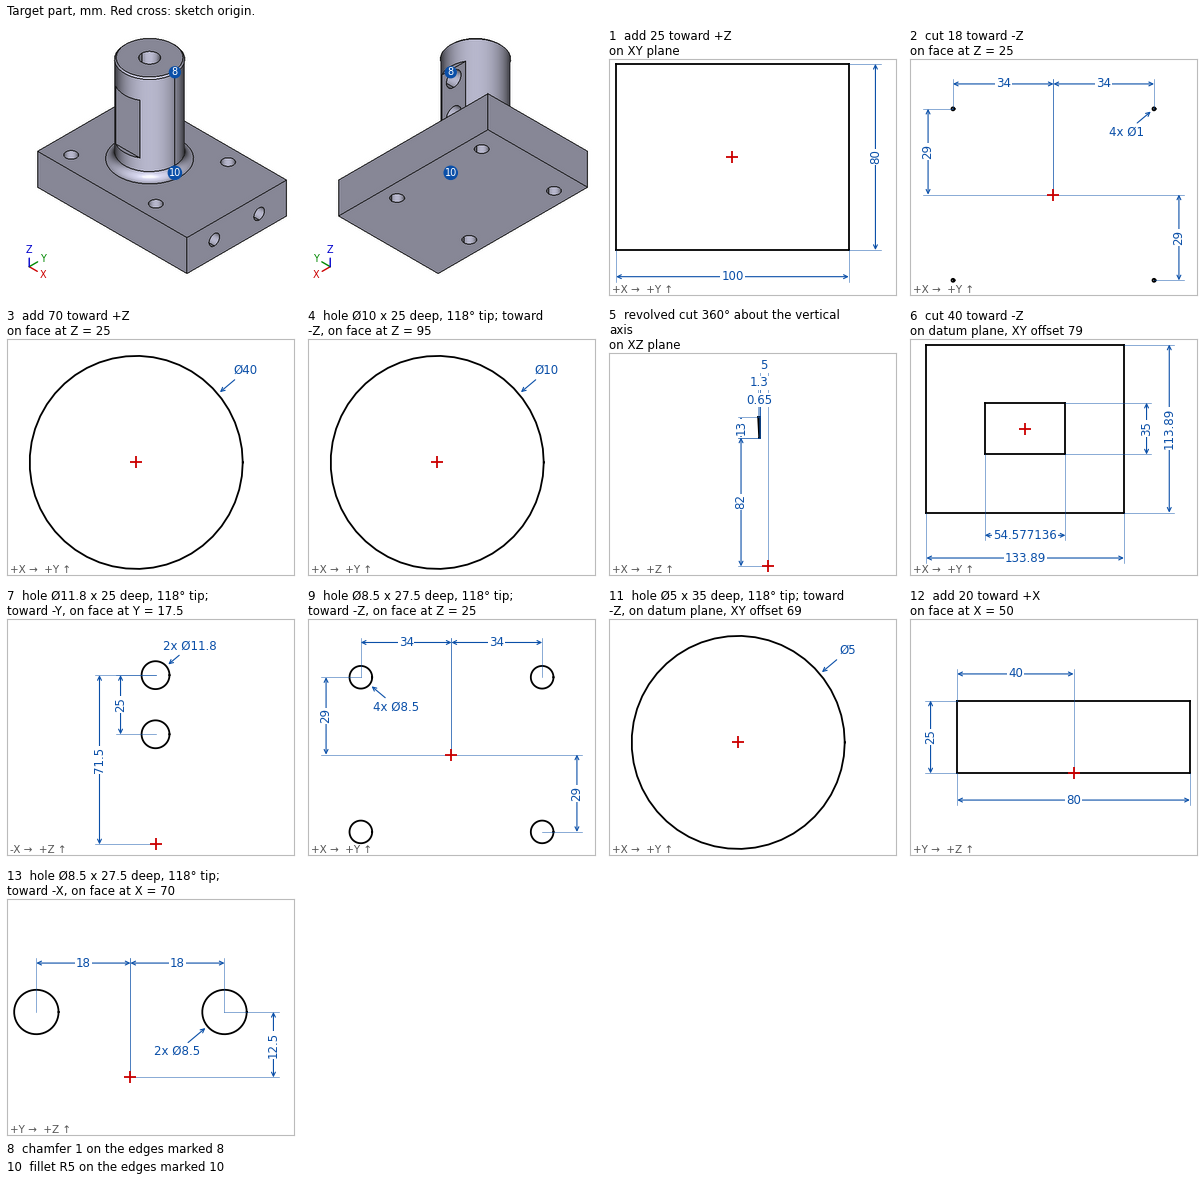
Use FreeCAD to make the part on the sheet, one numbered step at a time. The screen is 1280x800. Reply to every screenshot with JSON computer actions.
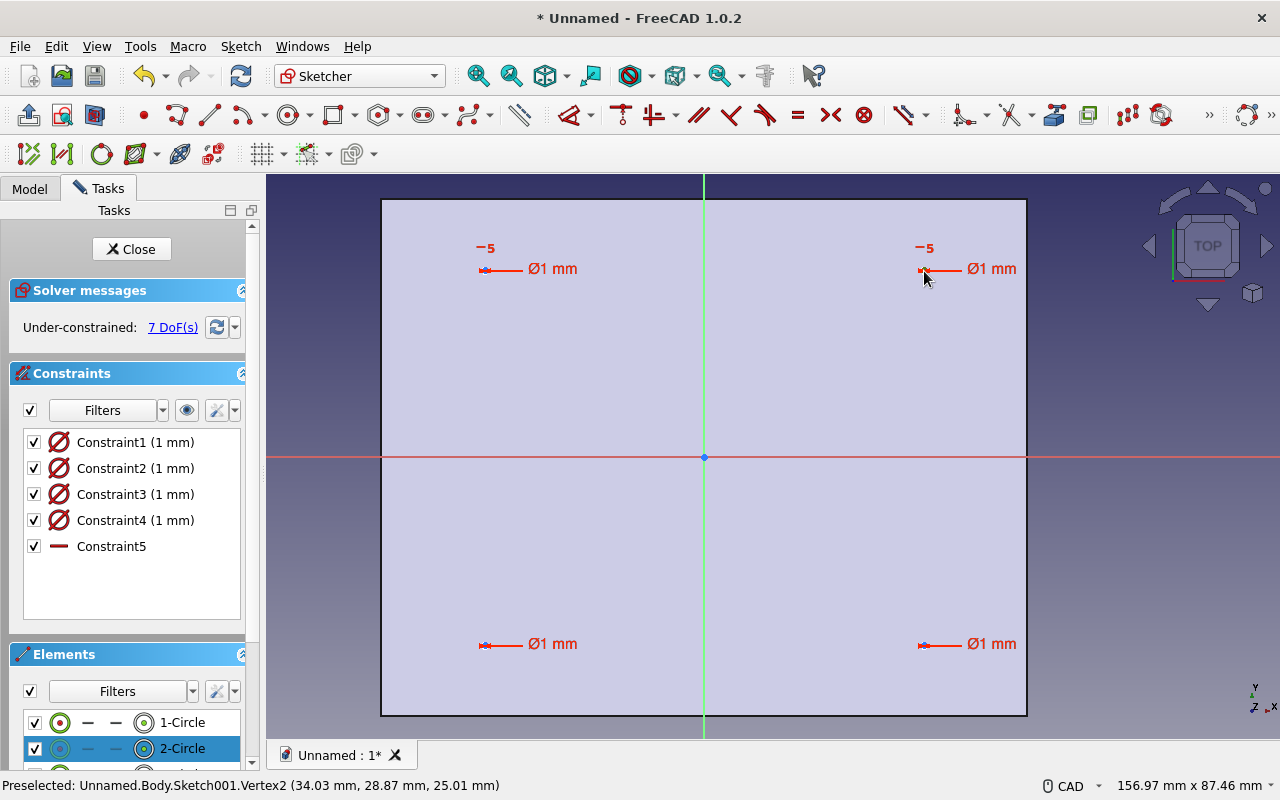
{"action": "left_click", "coordinate": [924, 646]}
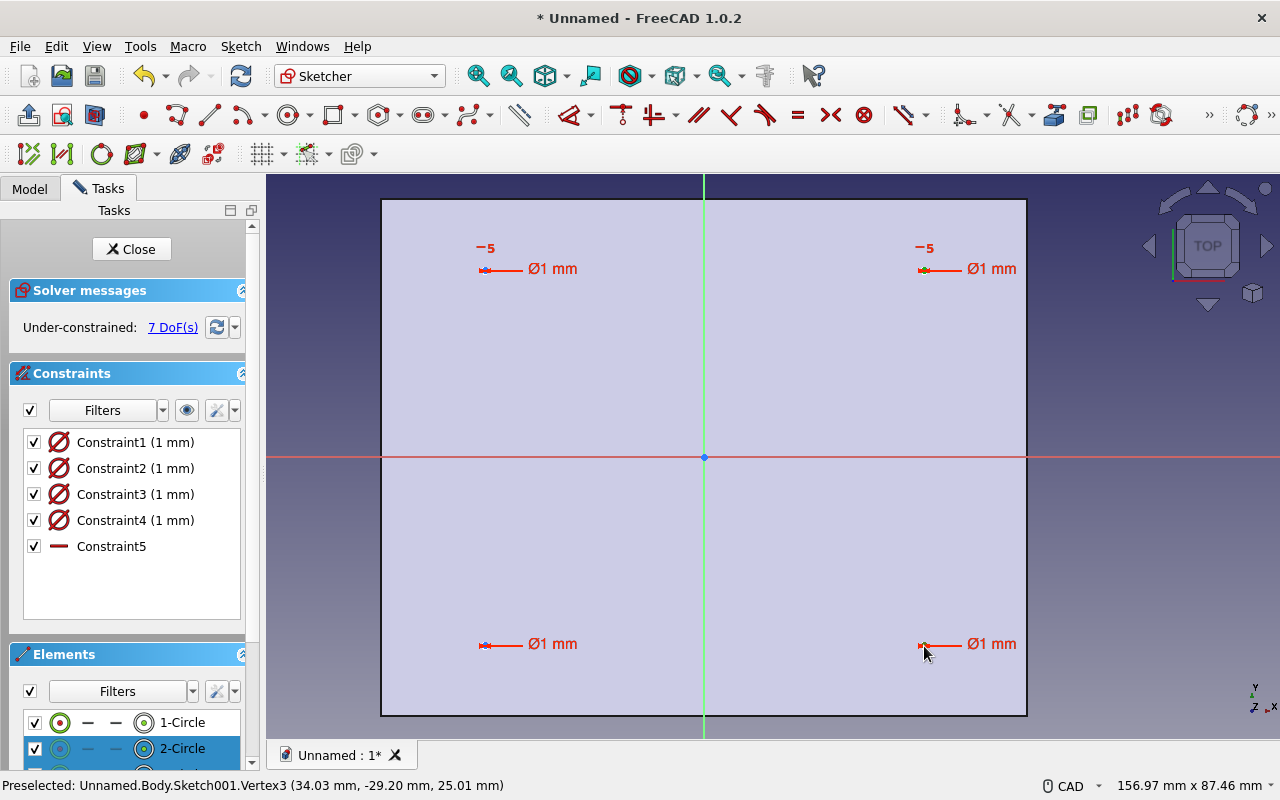
{"action": "key", "text": "v"}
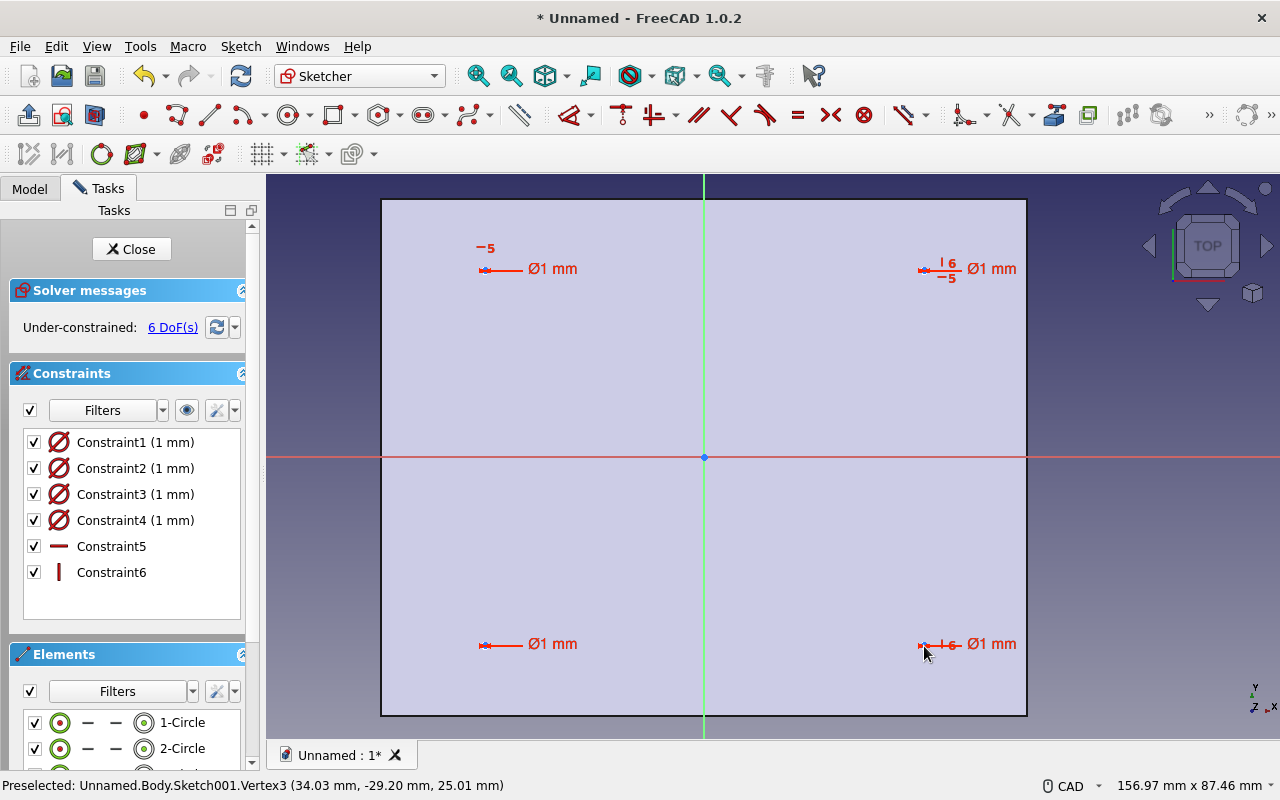
{"action": "left_click", "coordinate": [485, 271]}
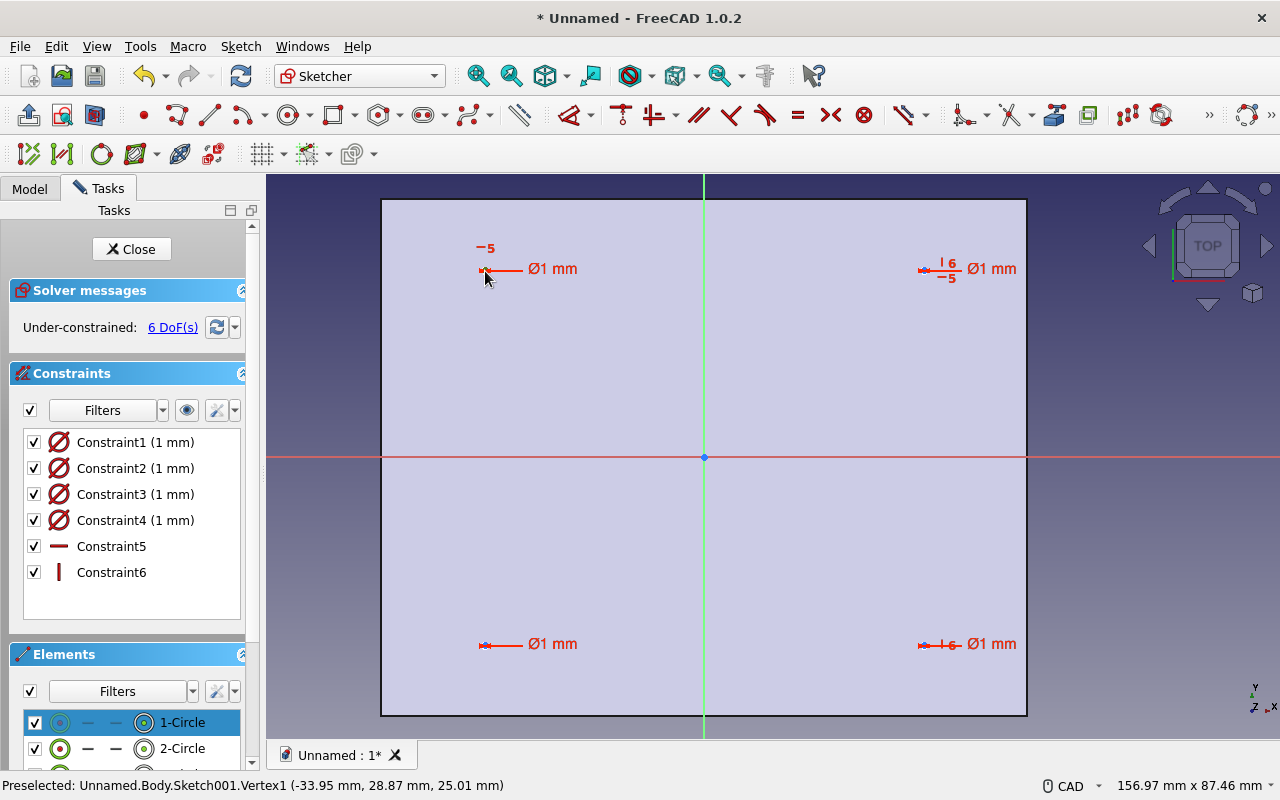
{"action": "left_click", "coordinate": [485, 646]}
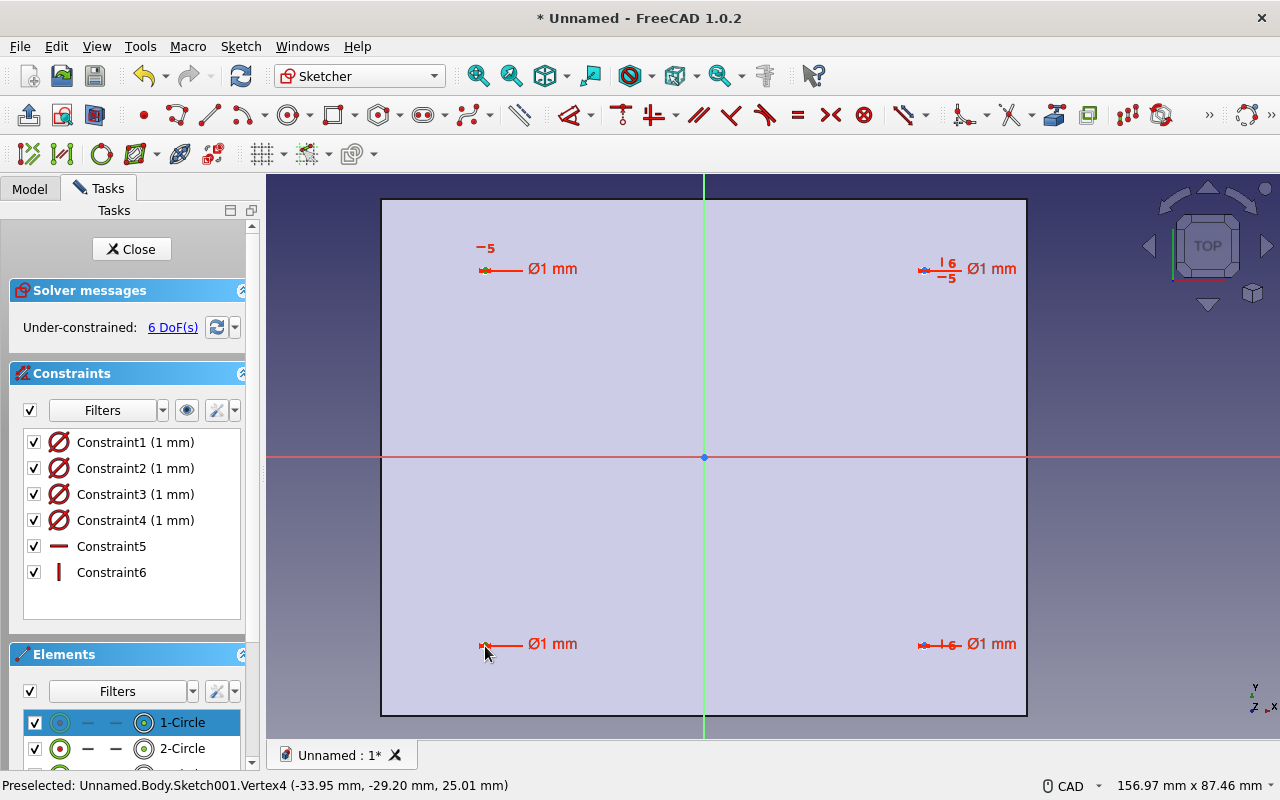
{"action": "key", "text": "v"}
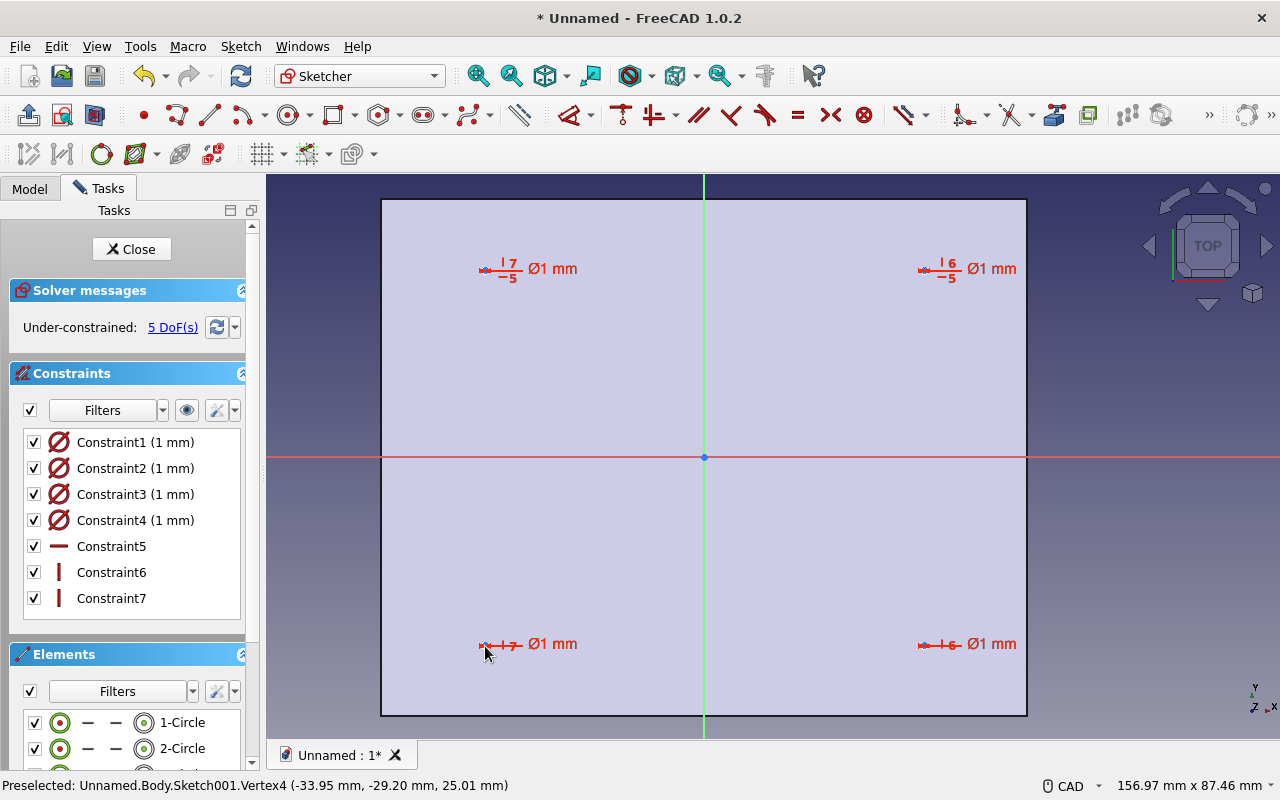
{"action": "left_click", "coordinate": [924, 646]}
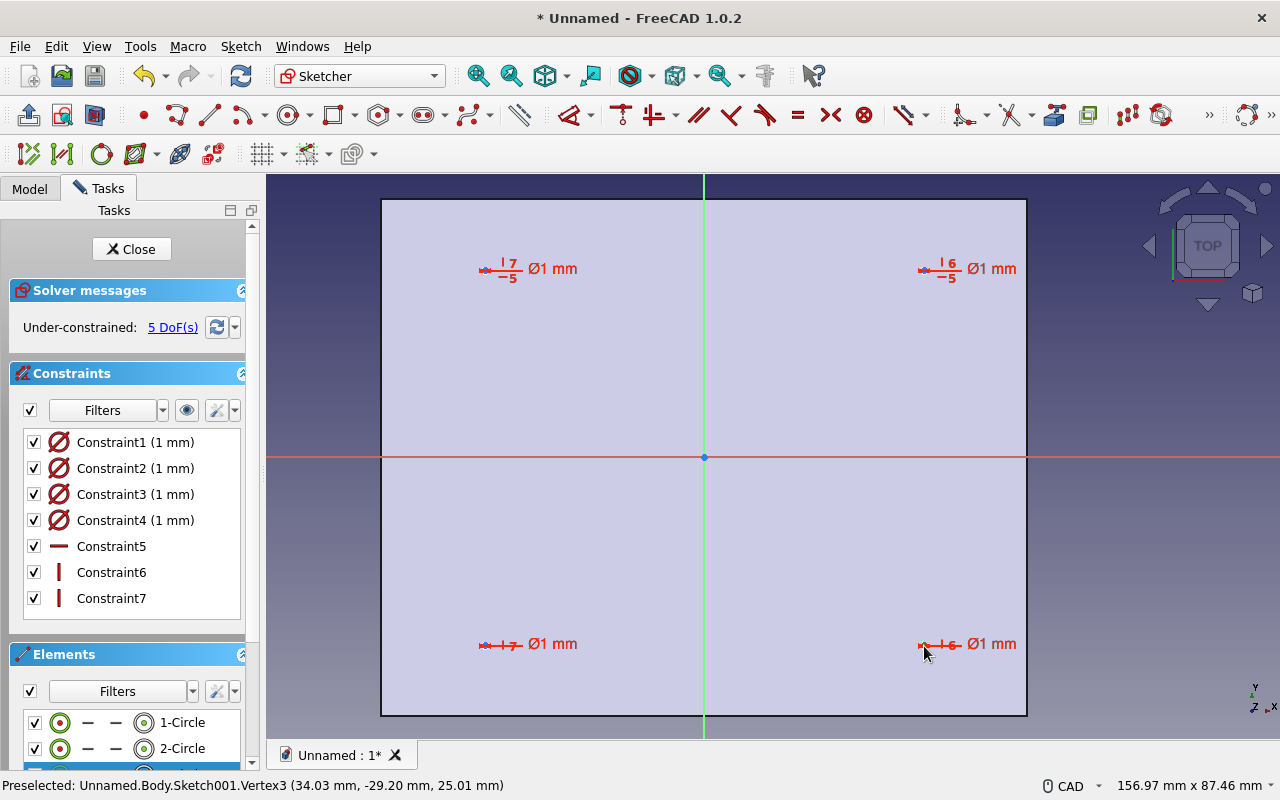
{"action": "left_click", "coordinate": [485, 646]}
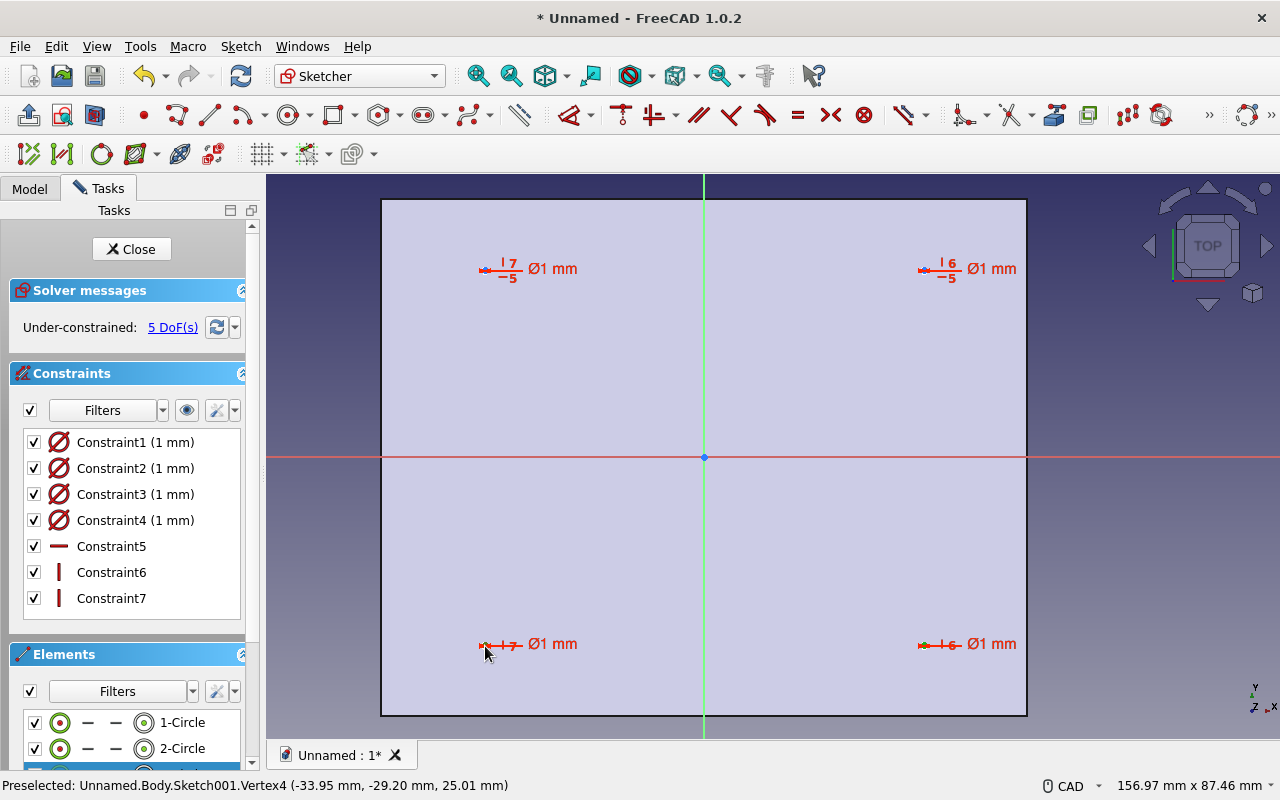
{"action": "key", "text": "h"}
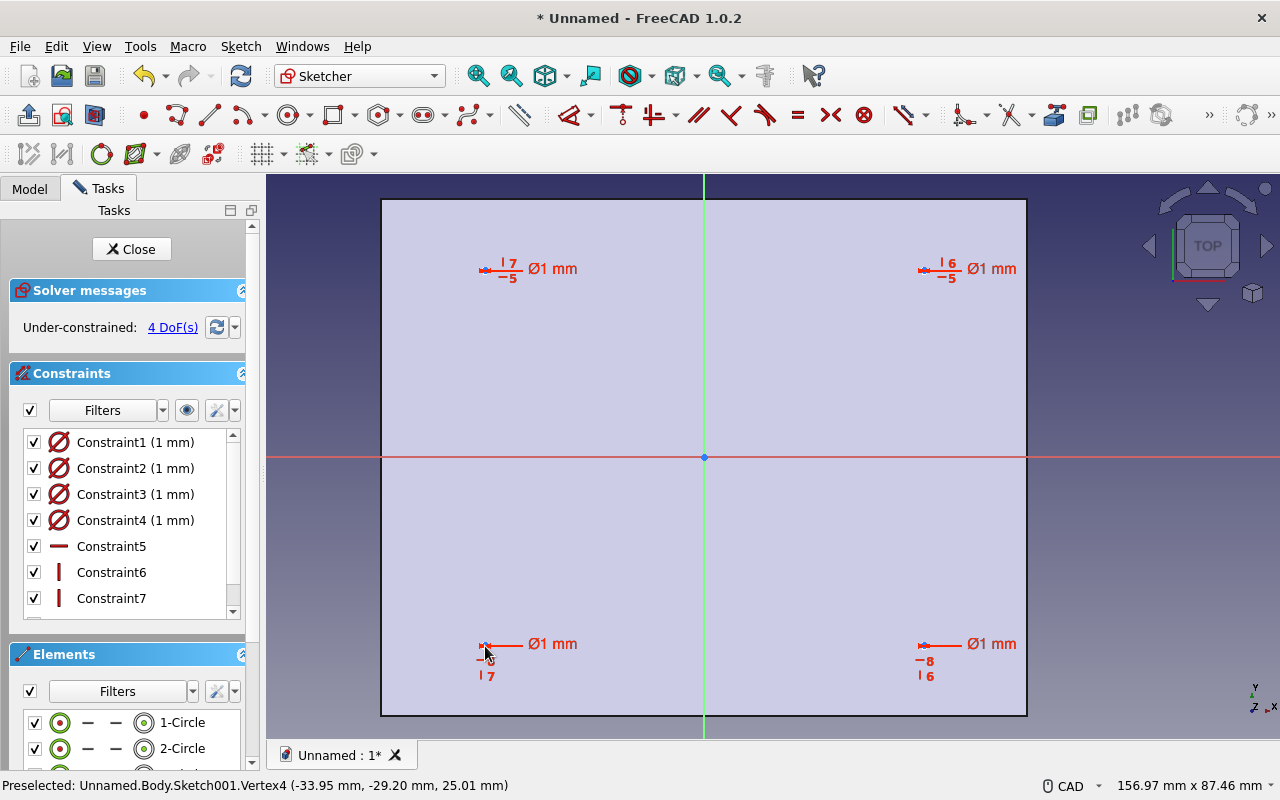
{"action": "left_click", "coordinate": [485, 271]}